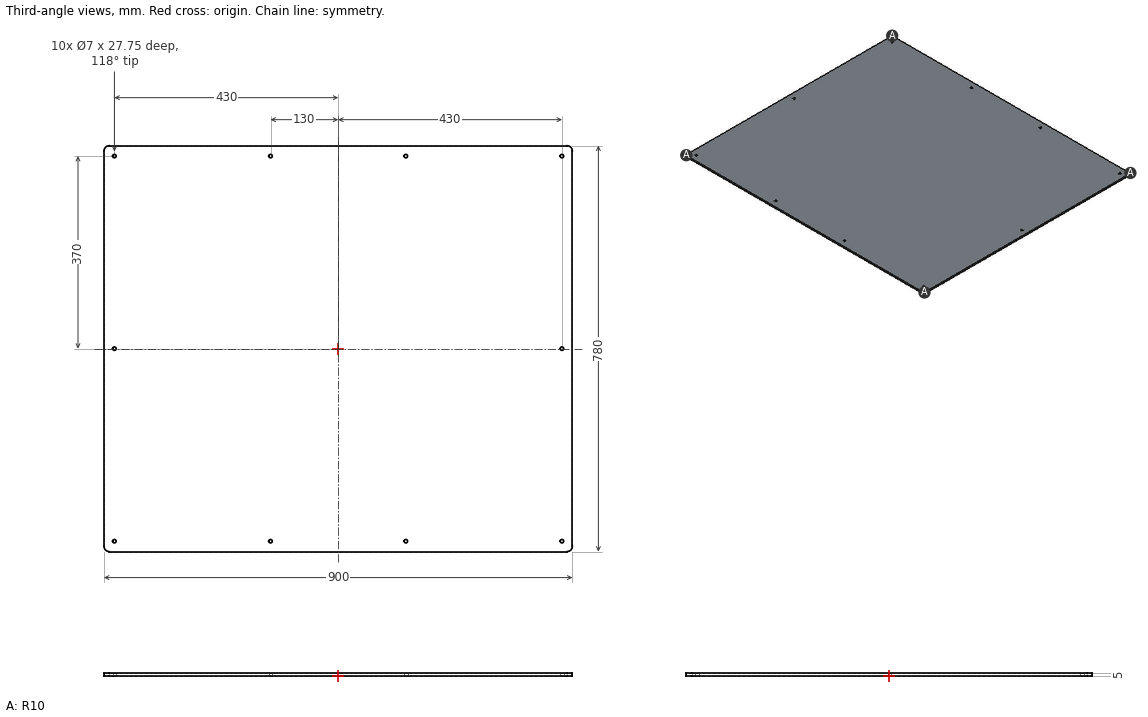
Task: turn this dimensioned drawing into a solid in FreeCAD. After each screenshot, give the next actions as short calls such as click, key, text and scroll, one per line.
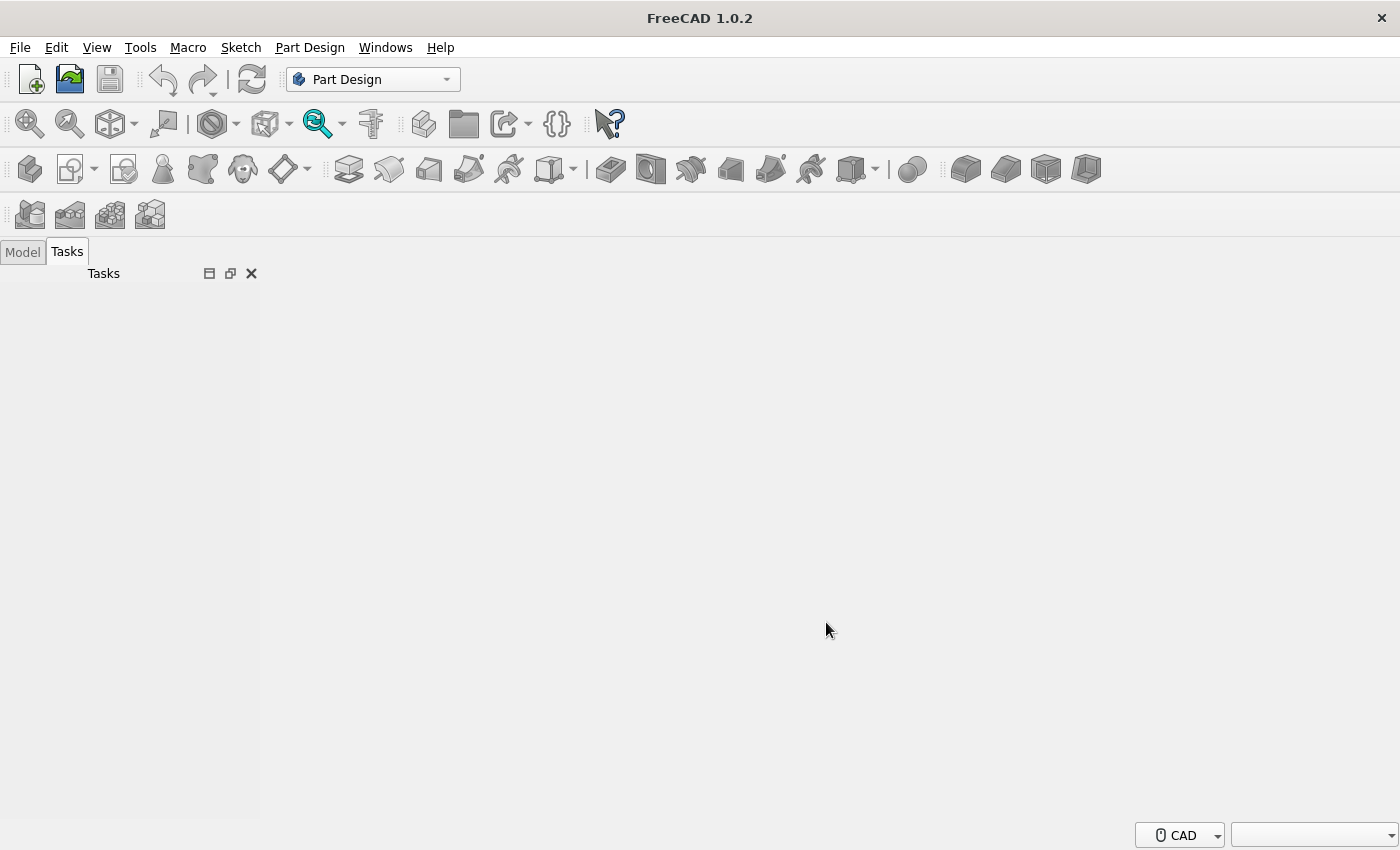
click(30, 80)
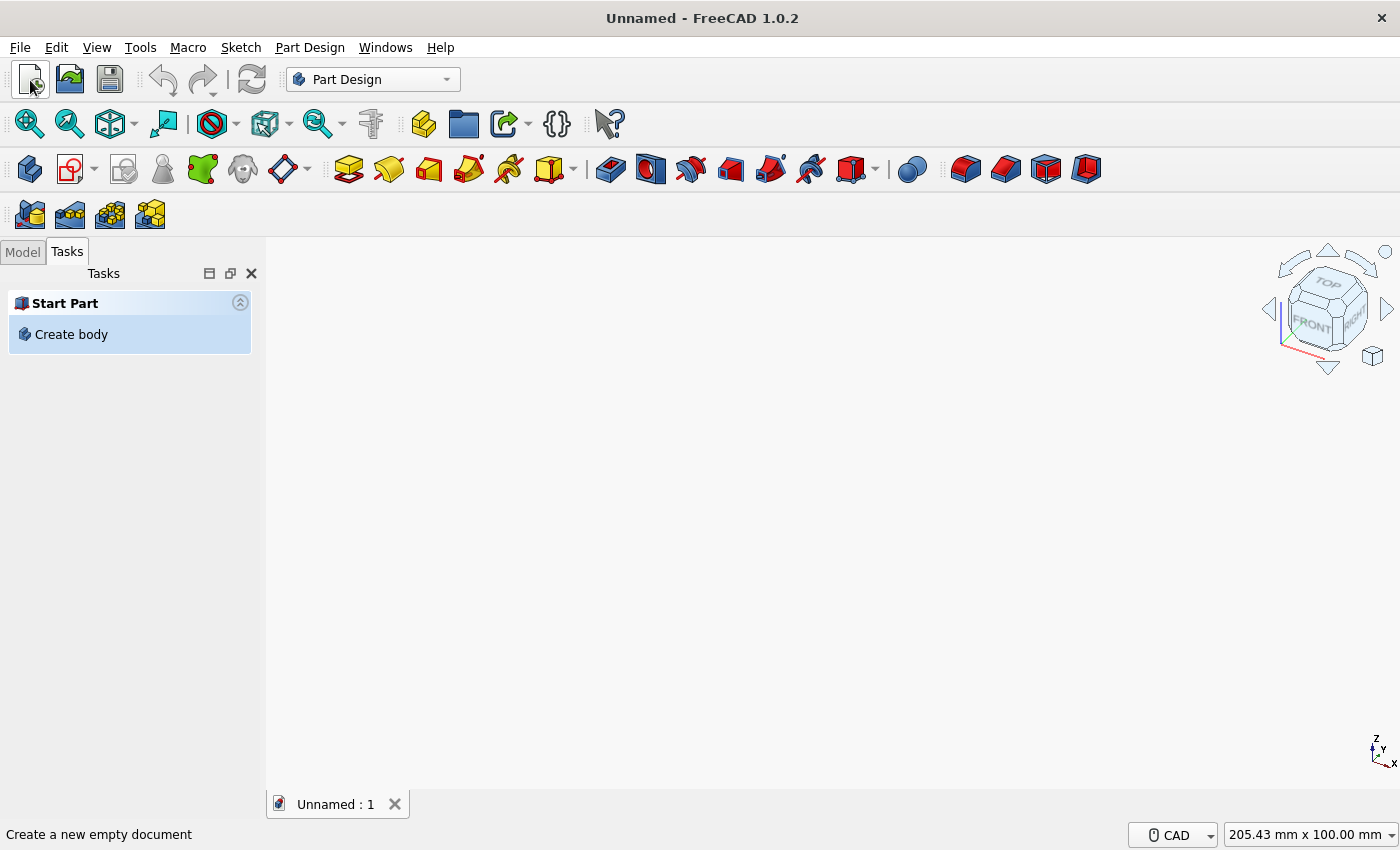
click(70, 170)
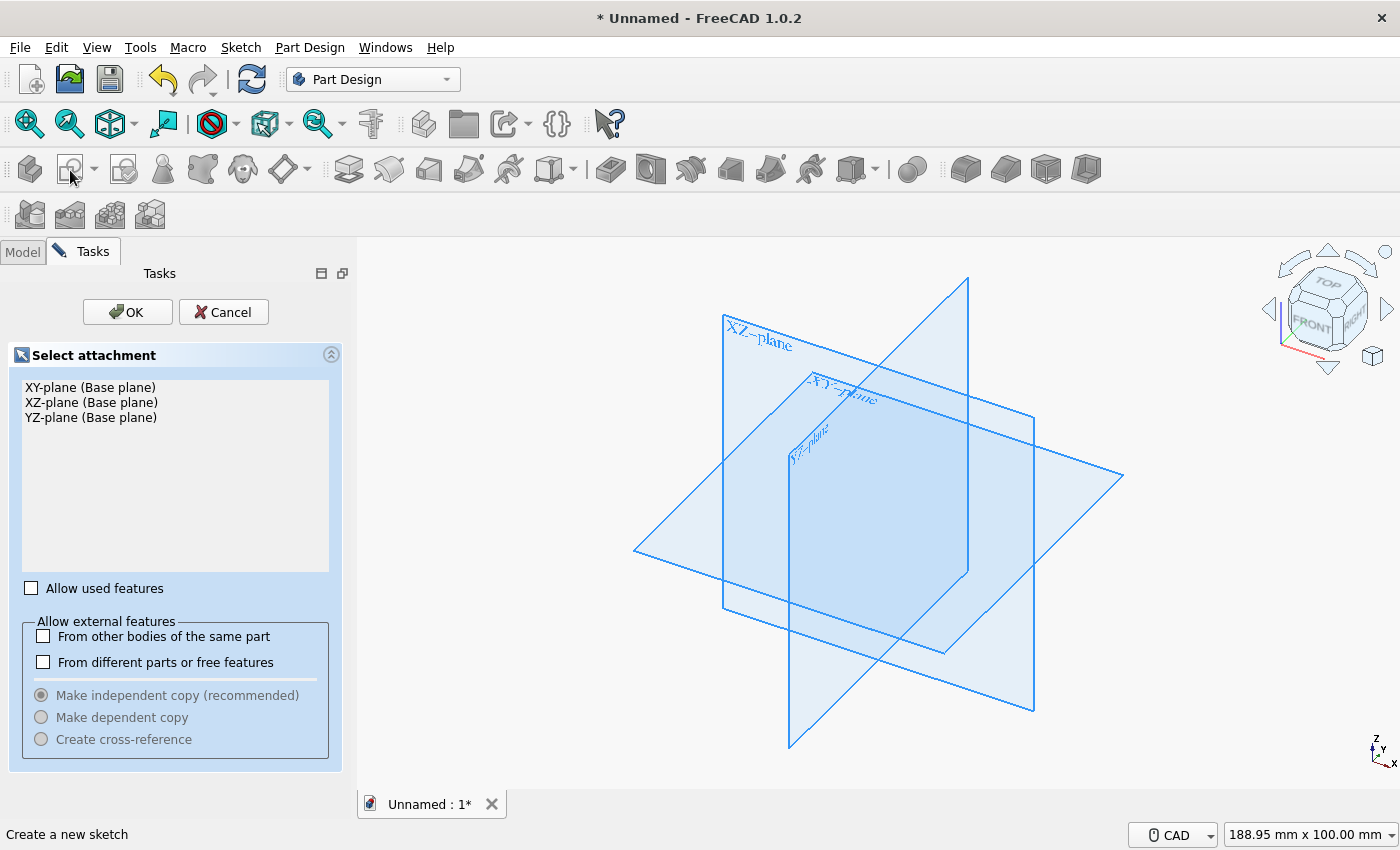
click(82, 388)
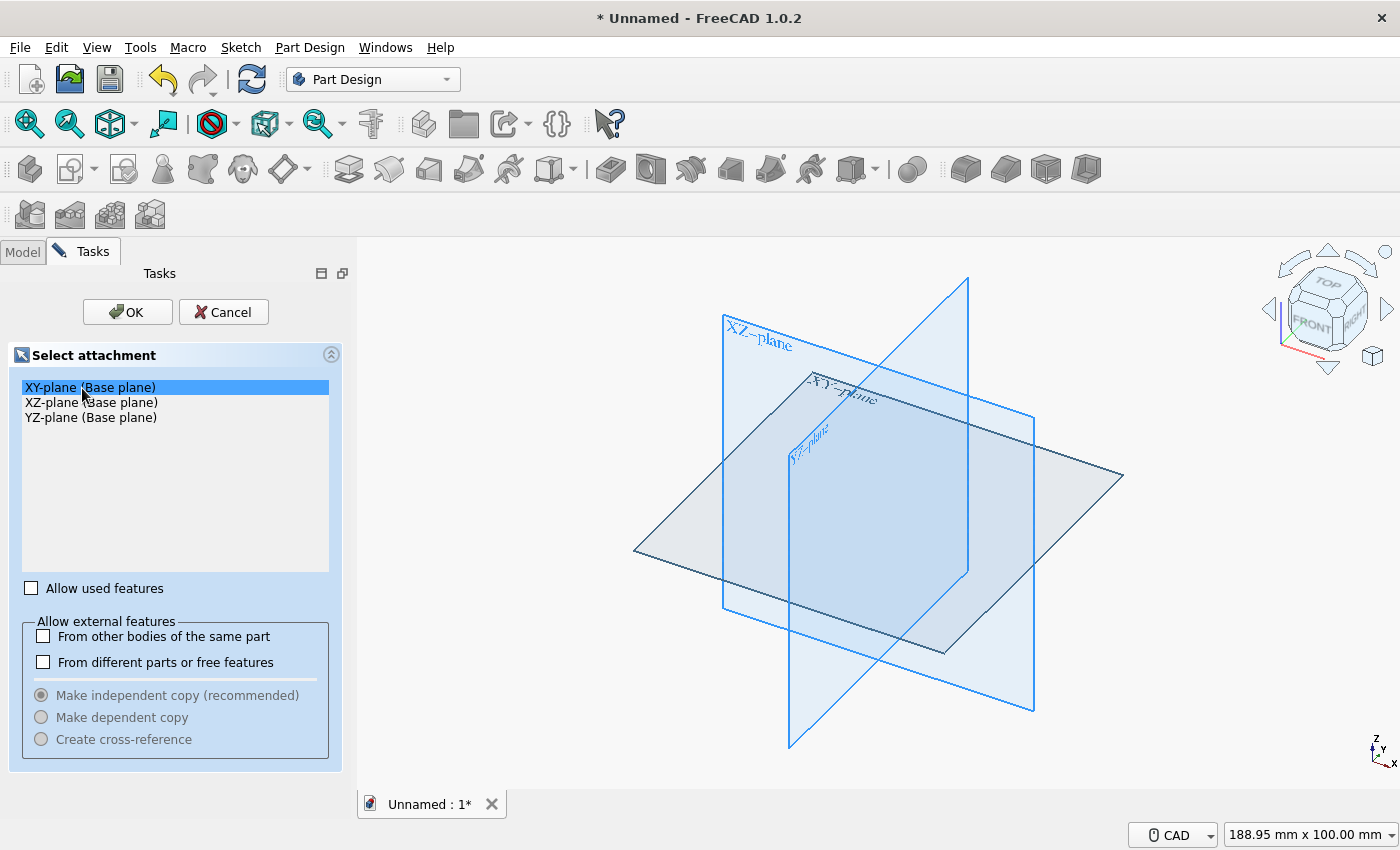
click(128, 312)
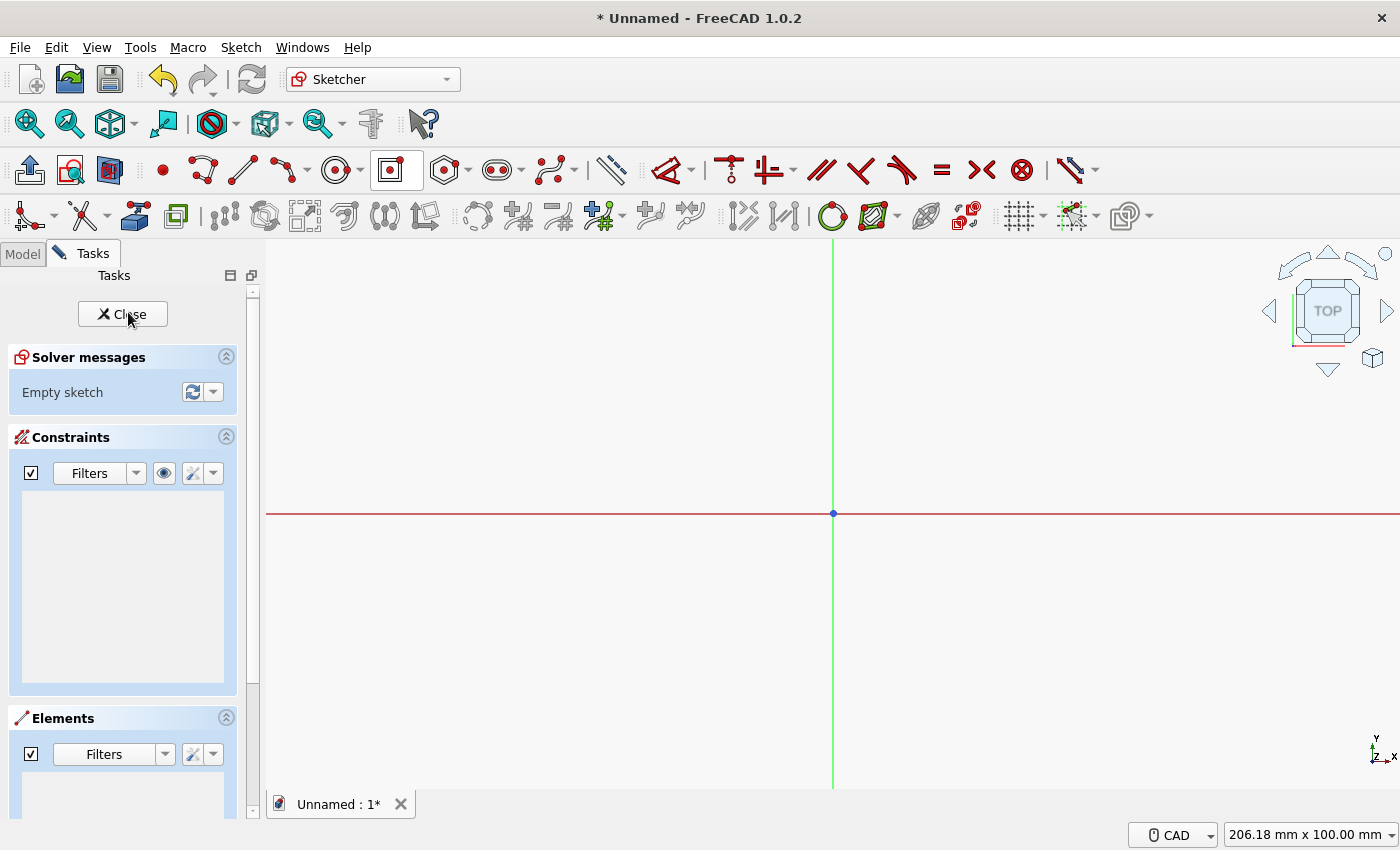
scroll(759, 514, down, 13)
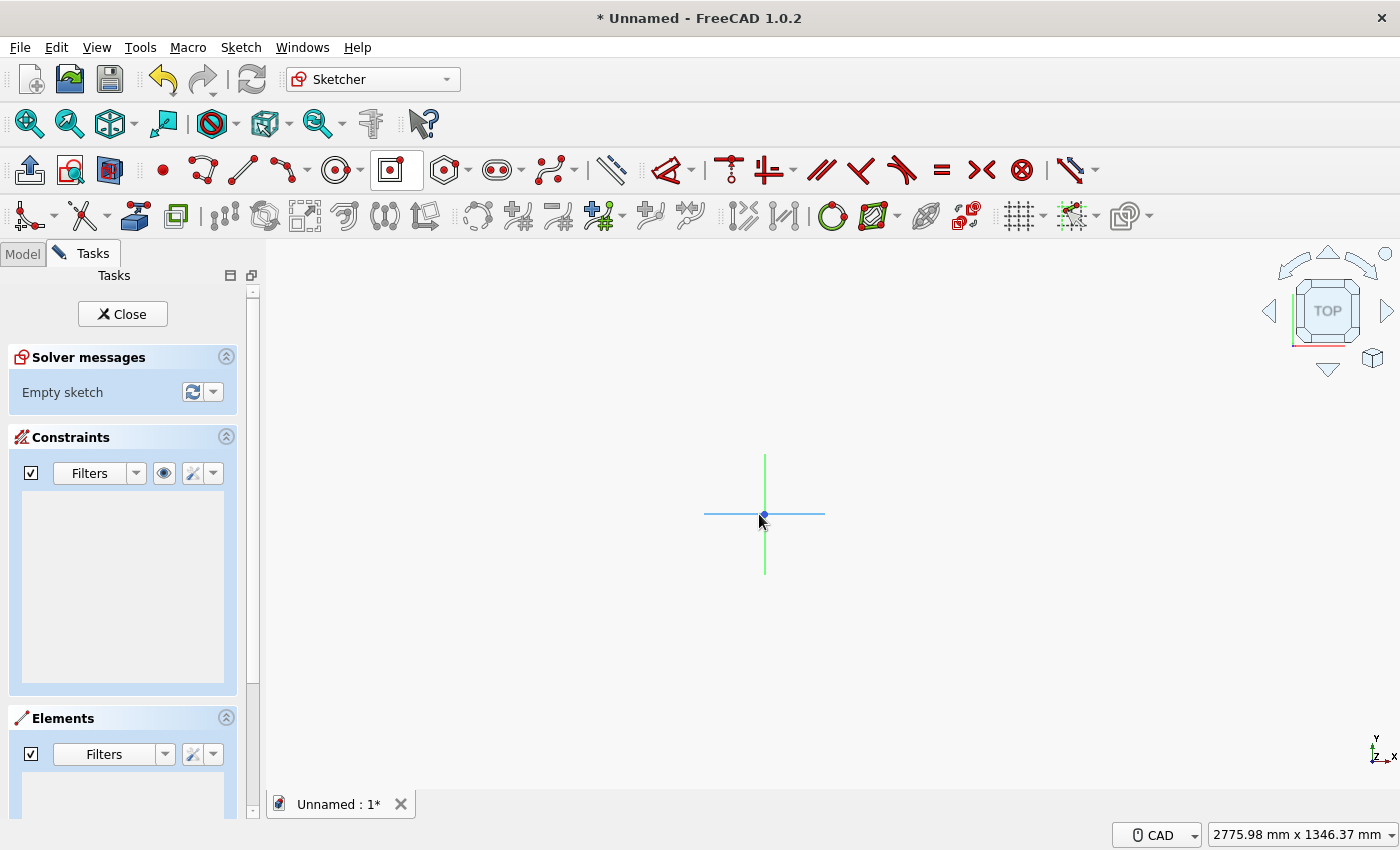
click(390, 170)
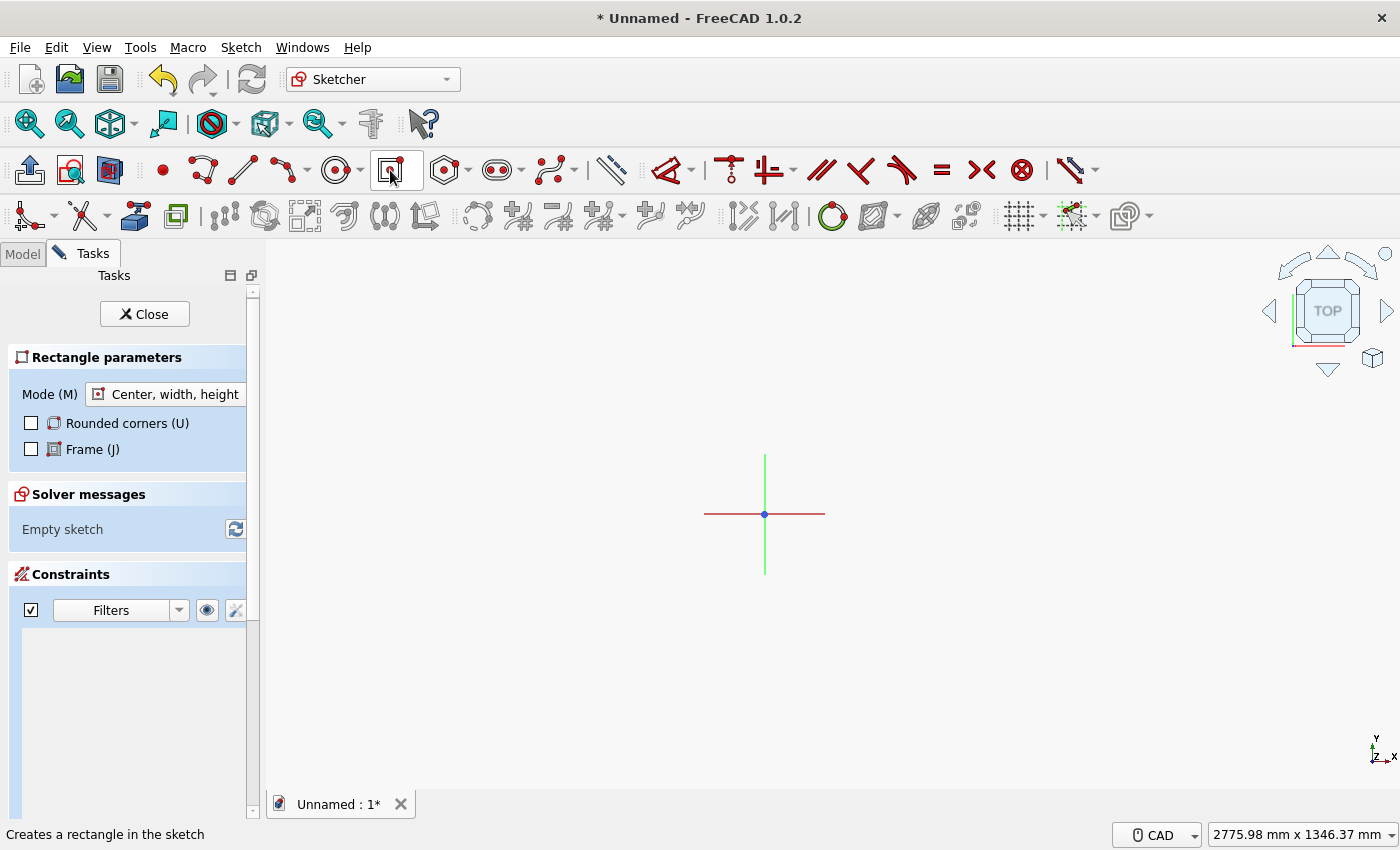
click(765, 514)
click(949, 355)
key(Escape)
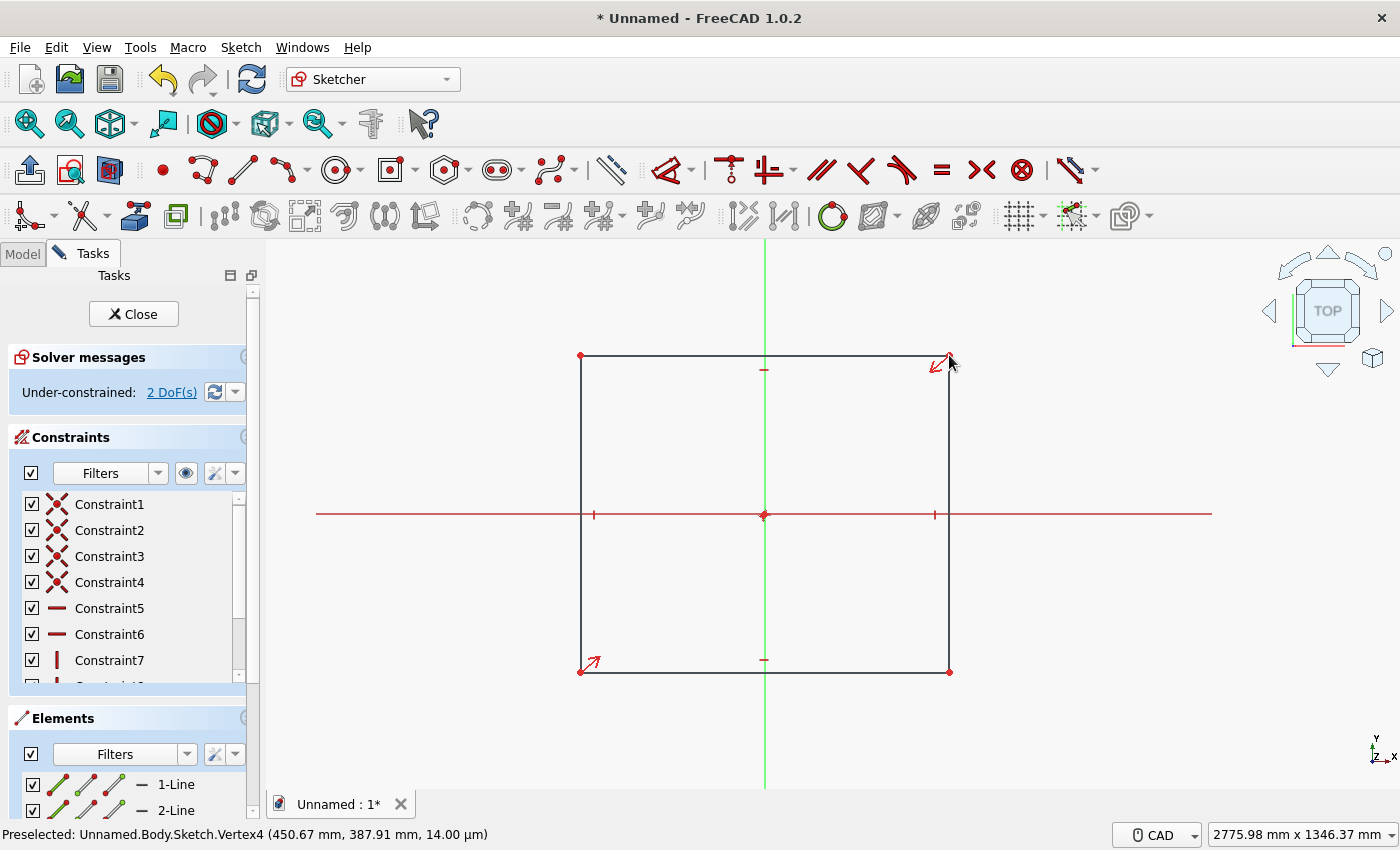
click(666, 170)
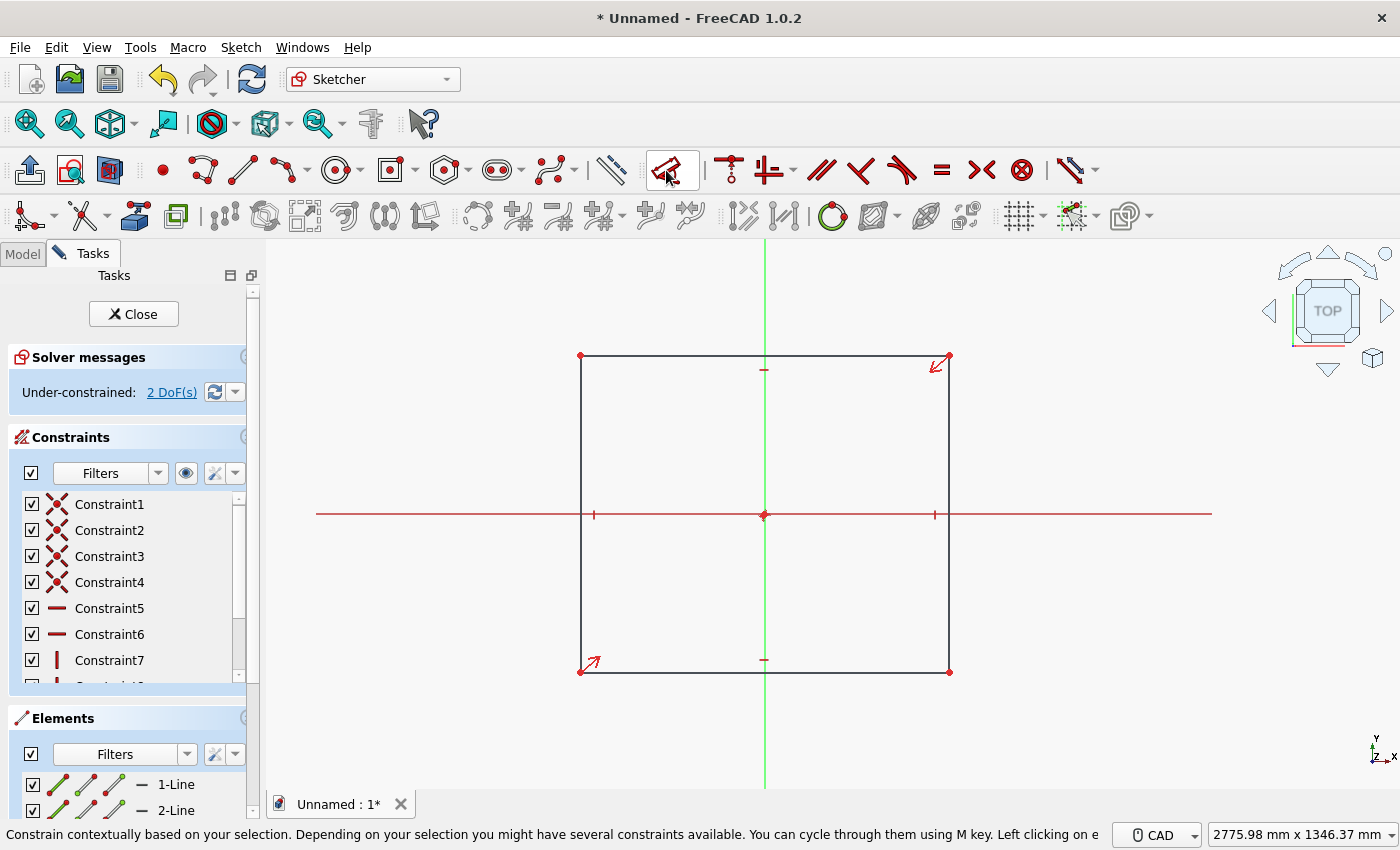
click(691, 673)
click(680, 707)